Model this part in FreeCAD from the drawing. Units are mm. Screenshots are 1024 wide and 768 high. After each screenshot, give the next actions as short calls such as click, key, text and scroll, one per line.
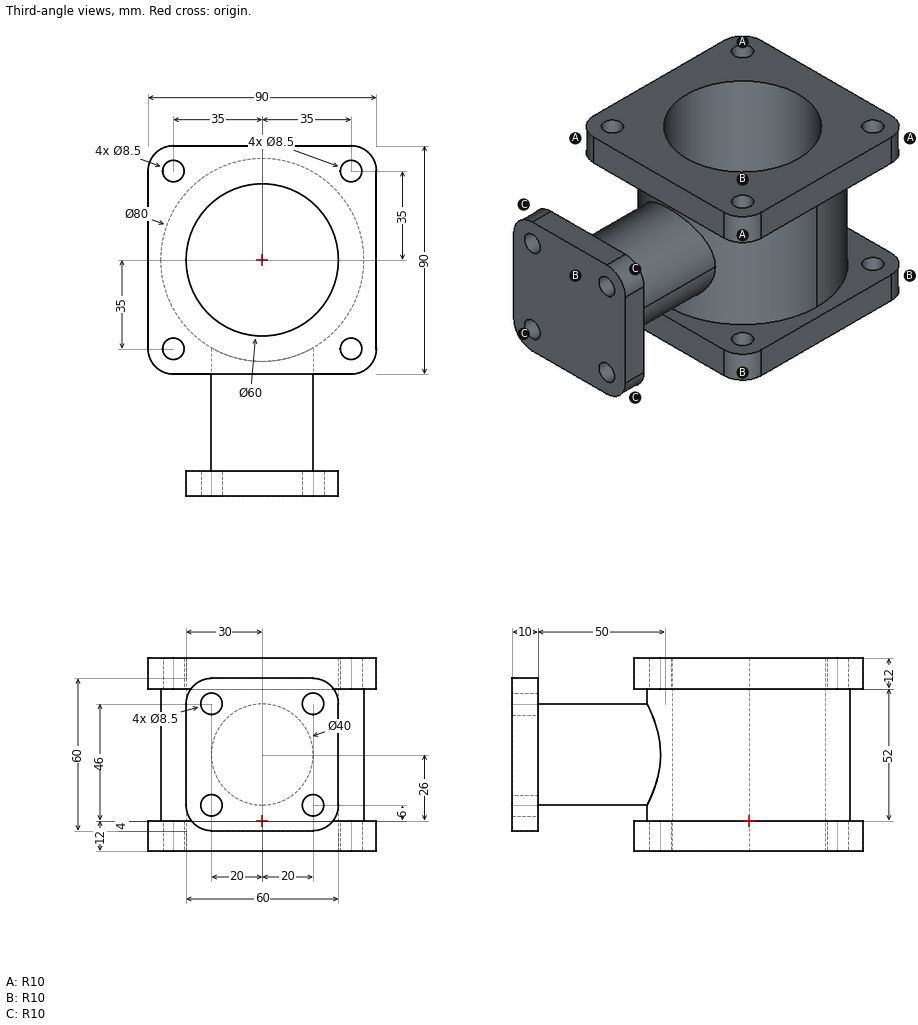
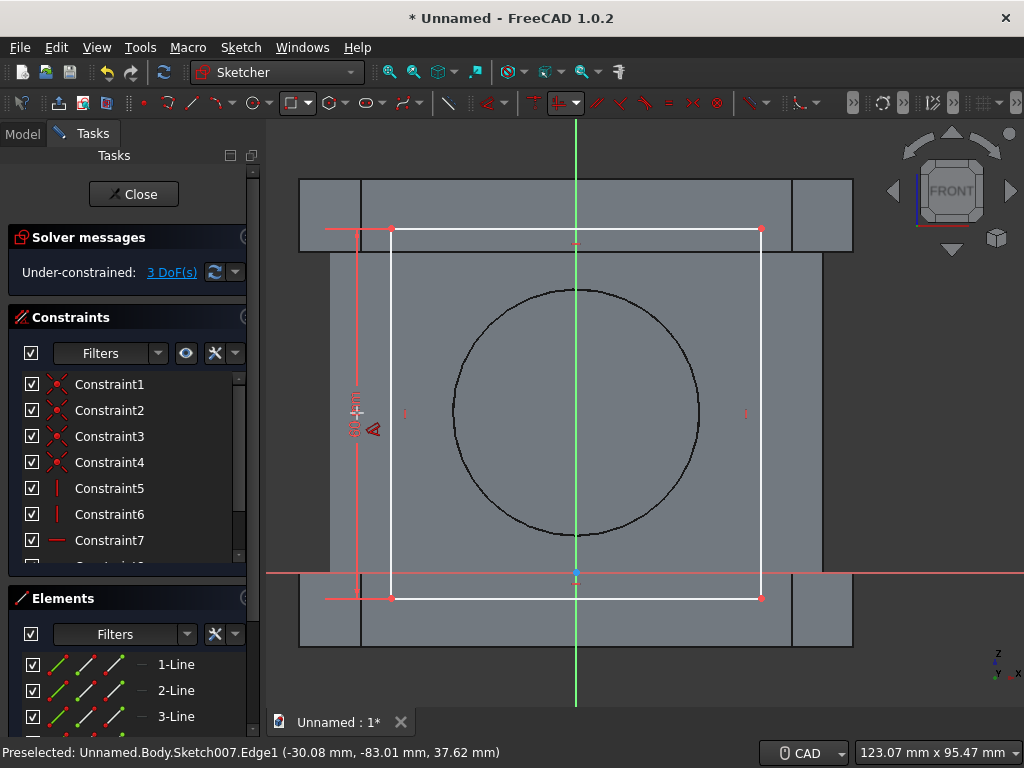
click(502, 599)
click(491, 633)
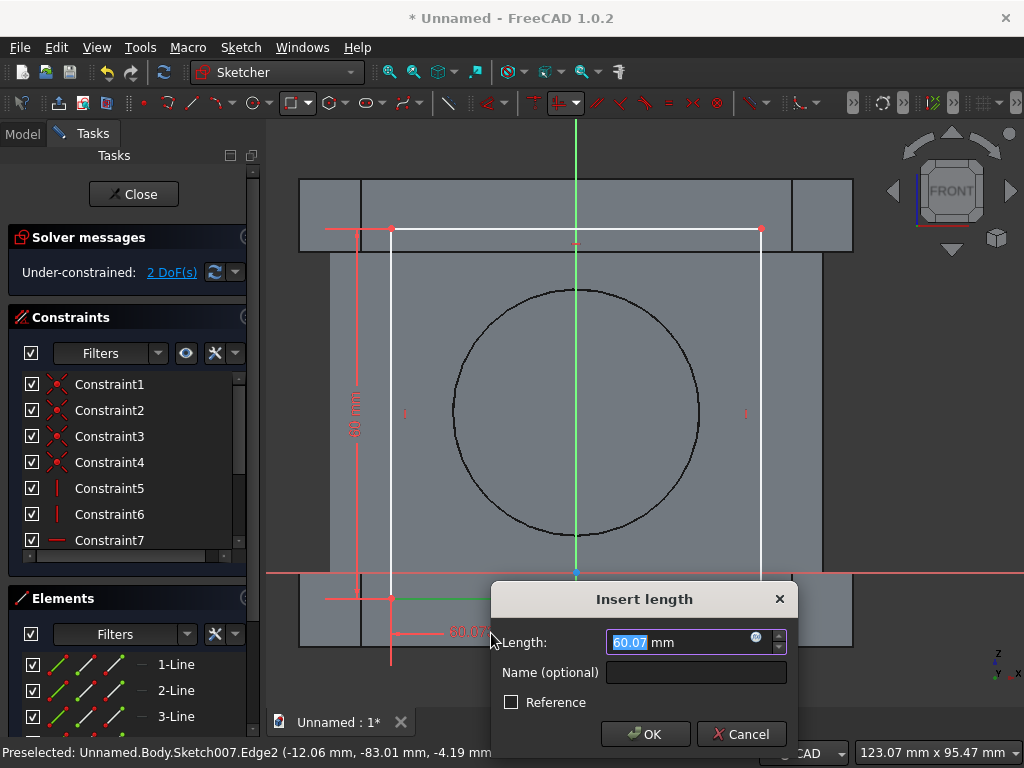
text(60)
key(Return)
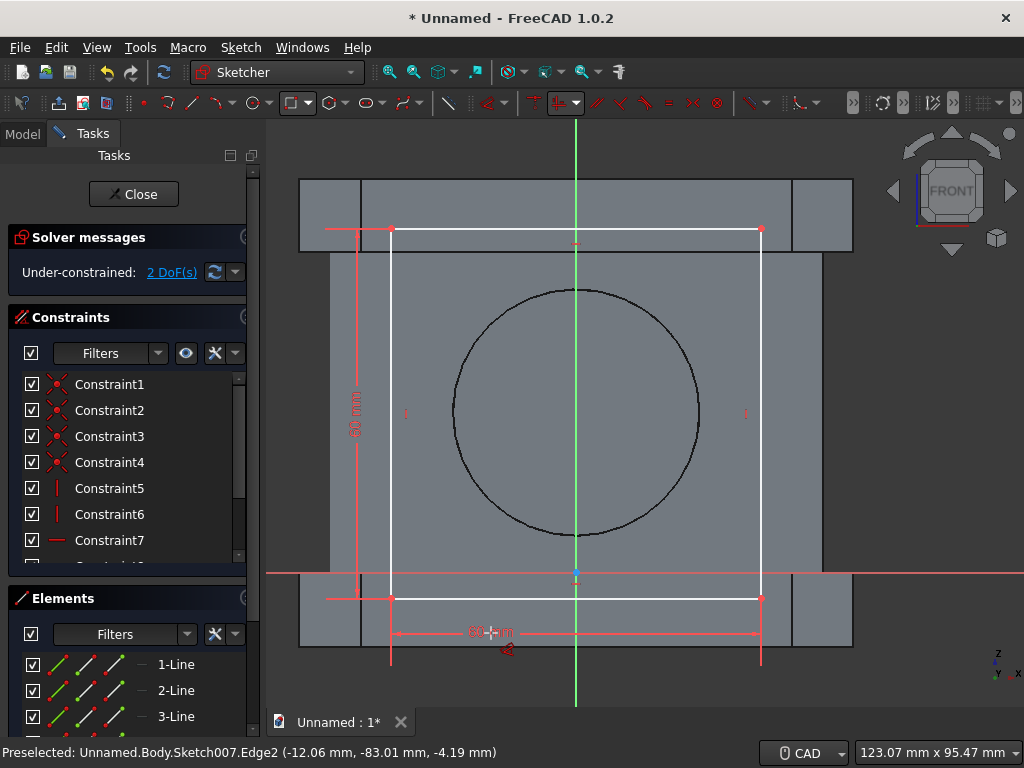
scroll(391, 599, up, 3)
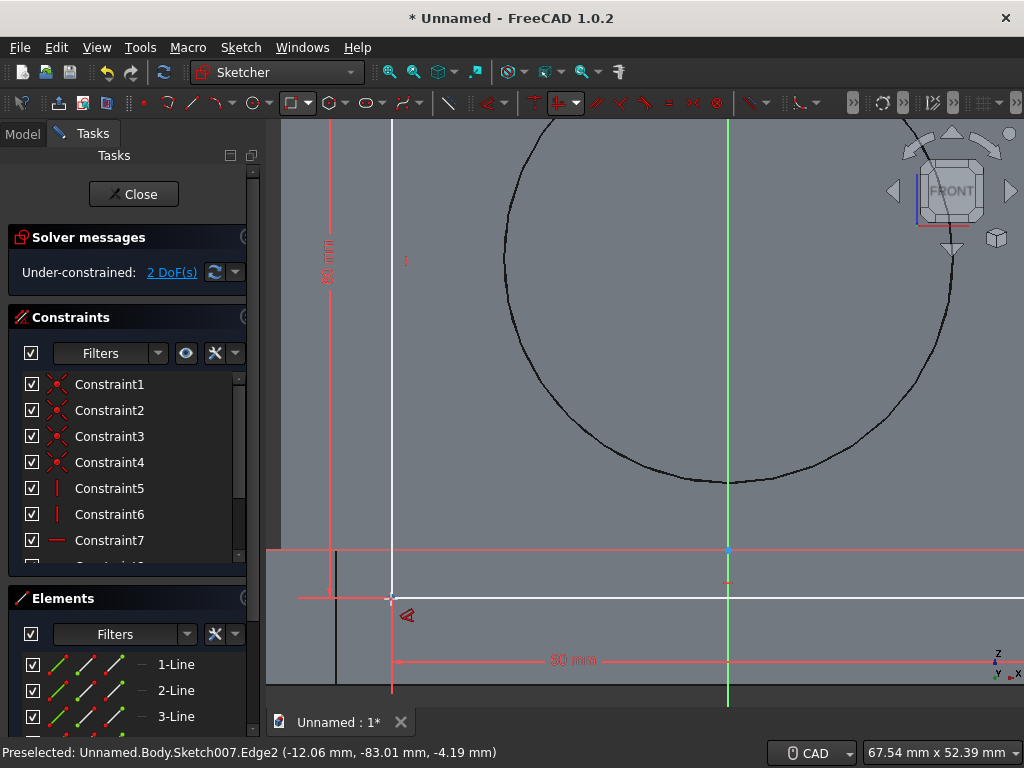
click(392, 598)
click(358, 574)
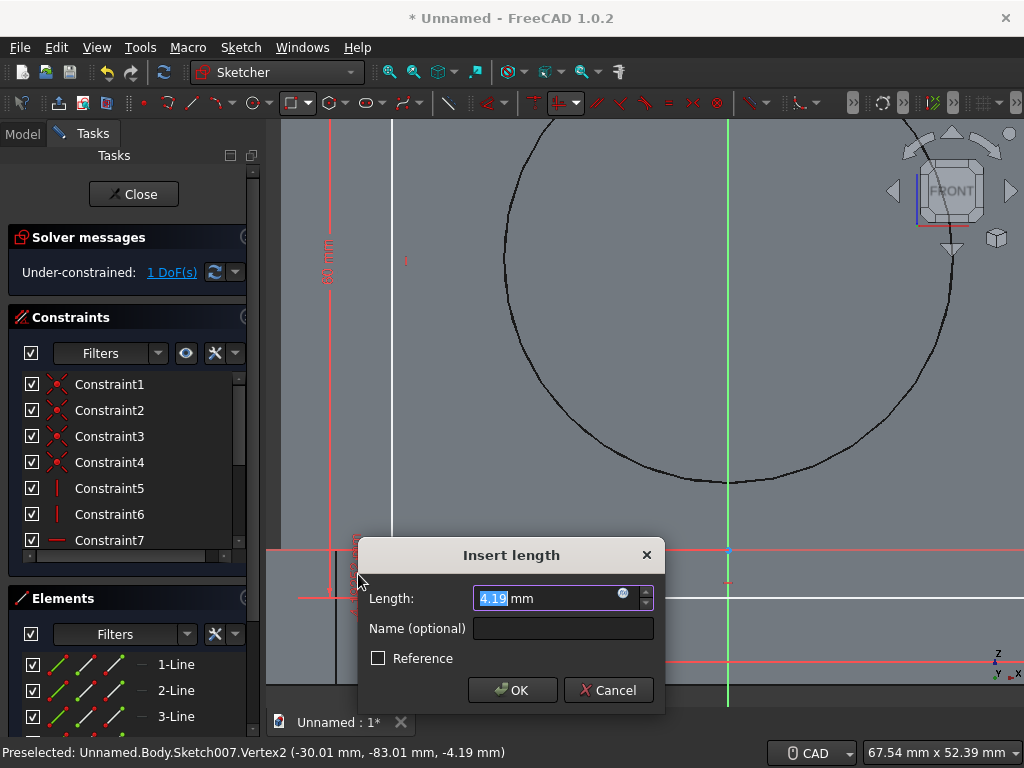
text(4)
key(Return)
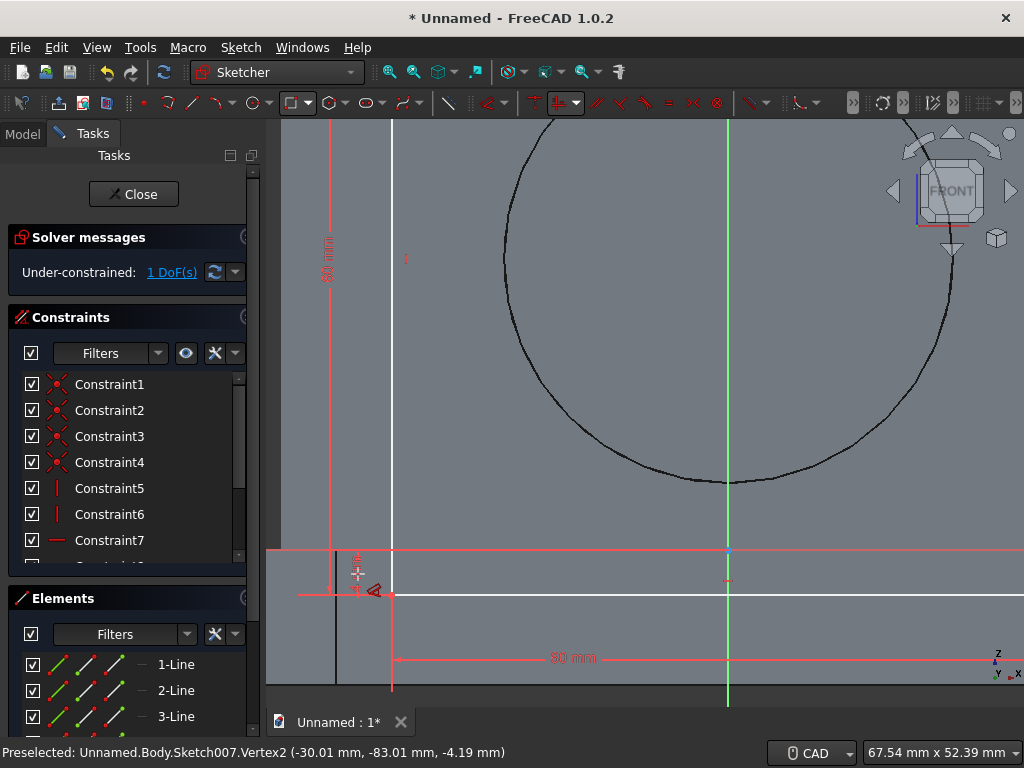
scroll(392, 601, down, 3)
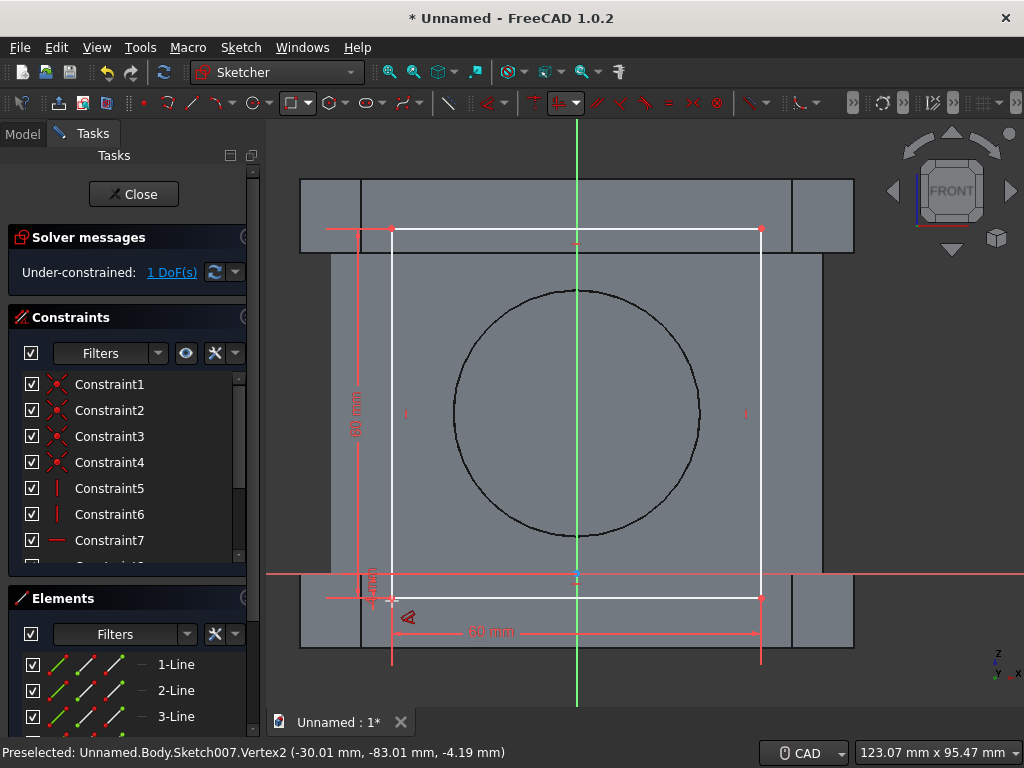
click(392, 229)
click(484, 195)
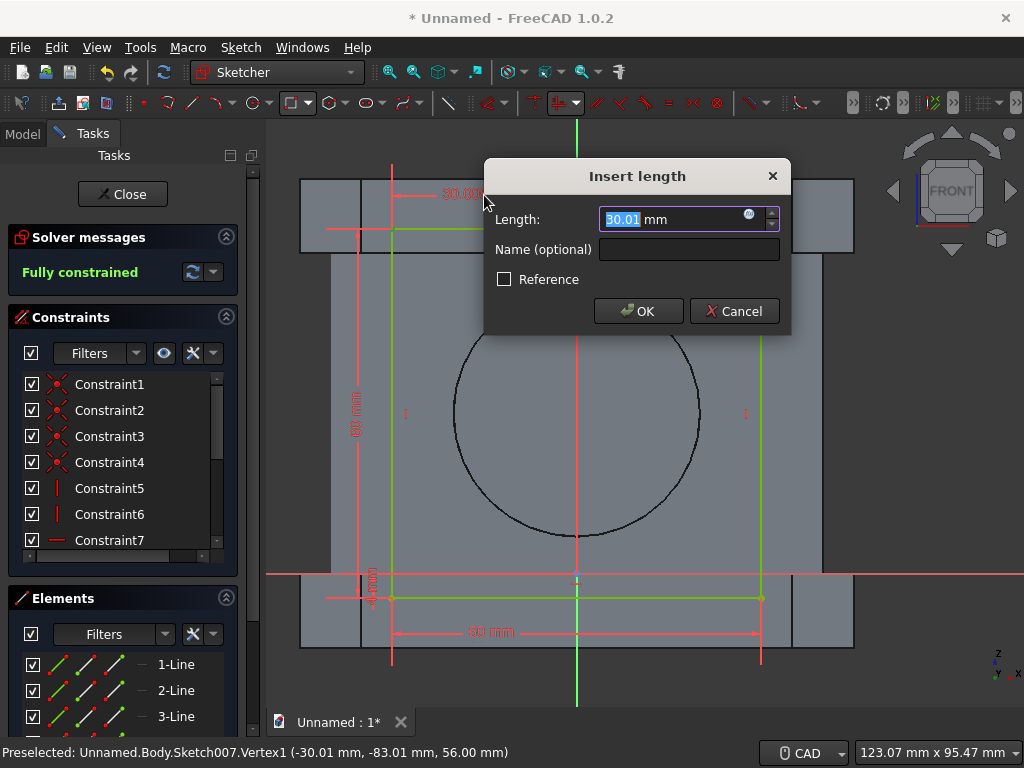
text(30)
key(Return)
key(Escape)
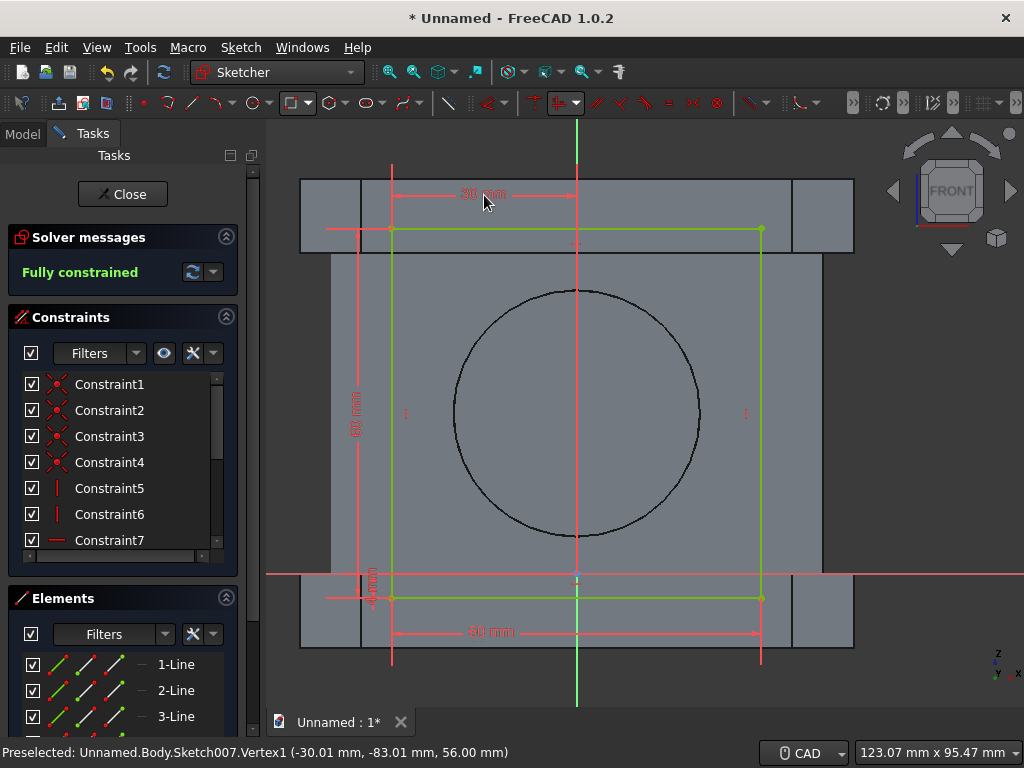
click(123, 194)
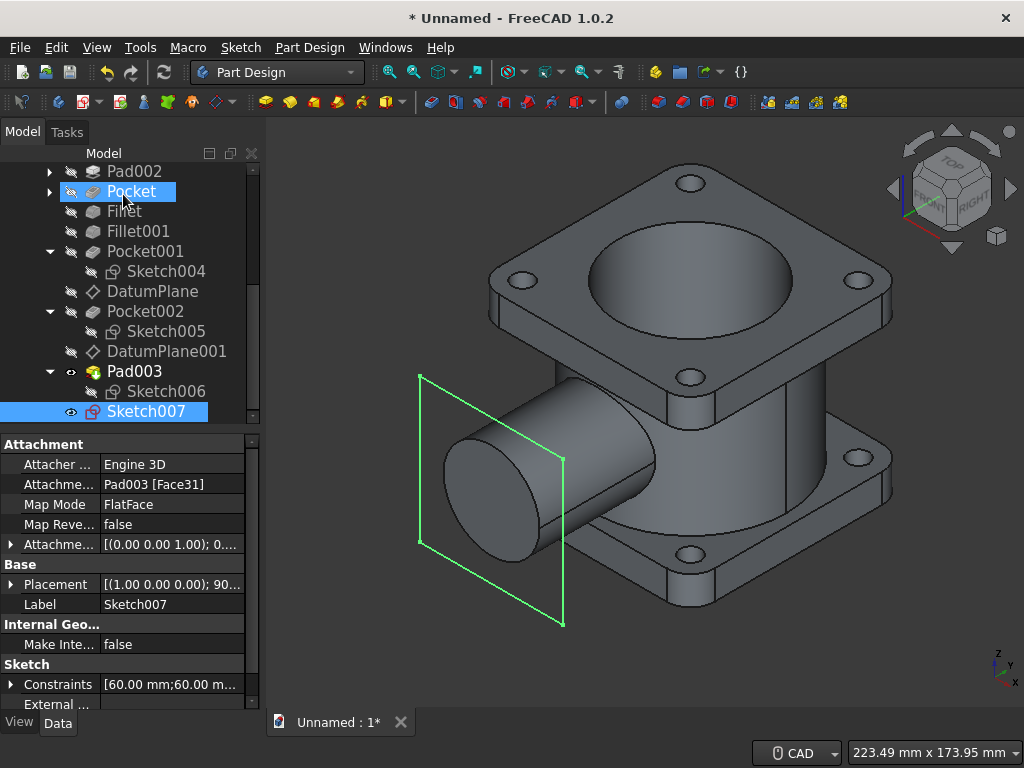
click(266, 102)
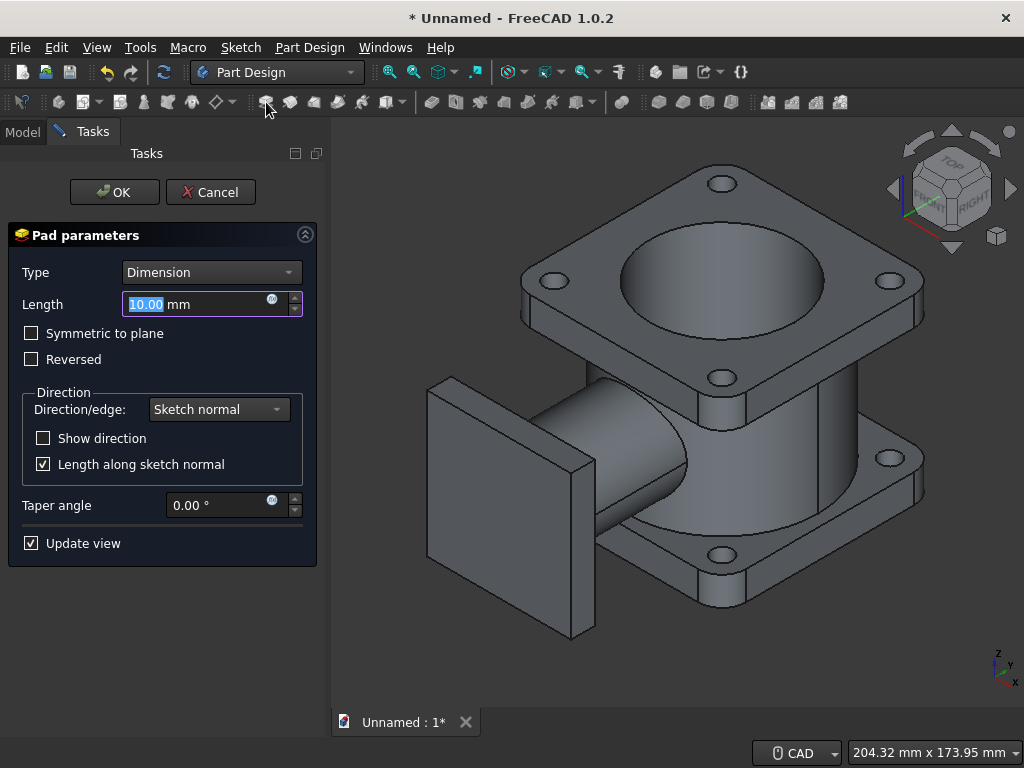
text(10)
key(Tab)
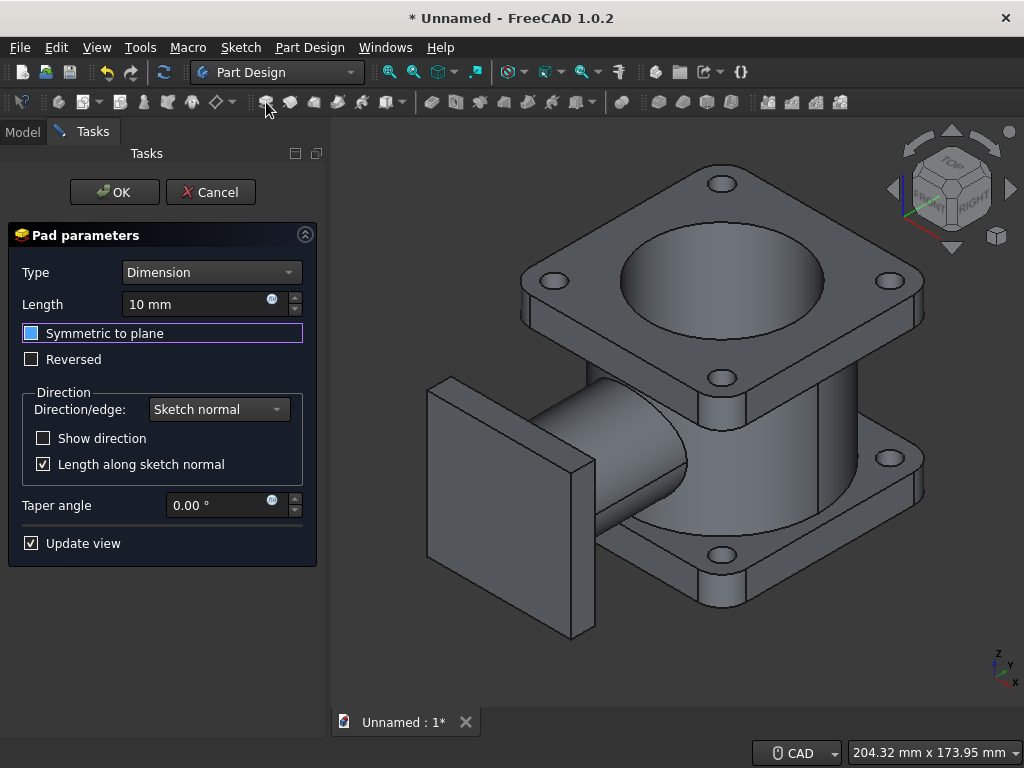
click(115, 192)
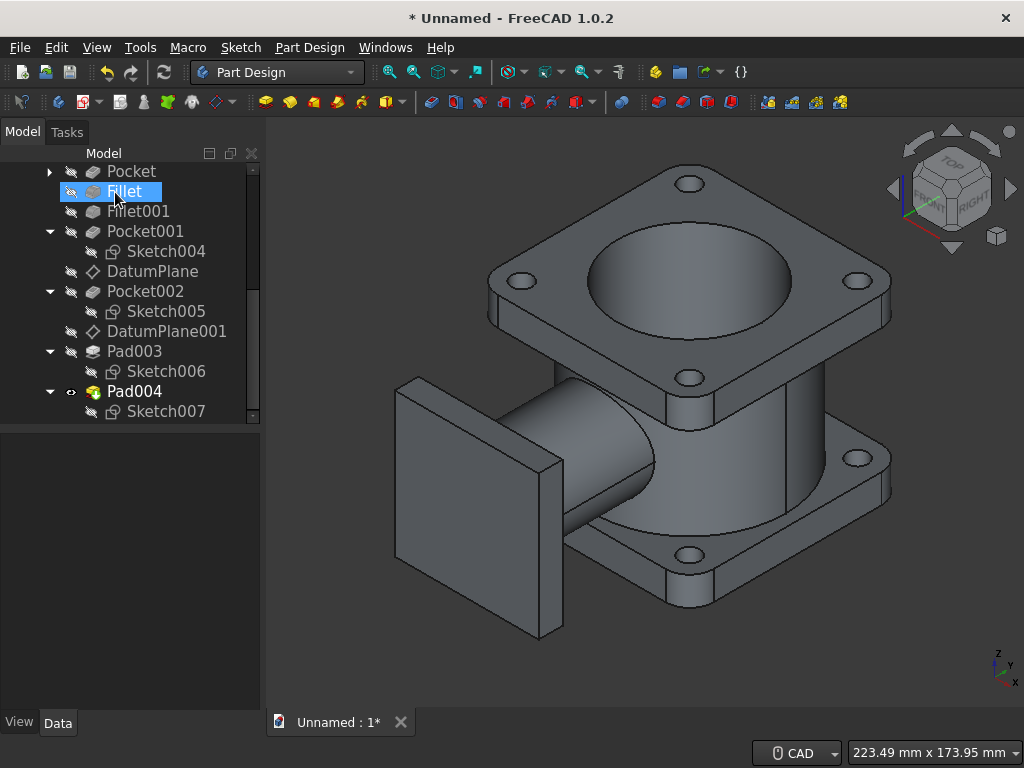
click(551, 466)